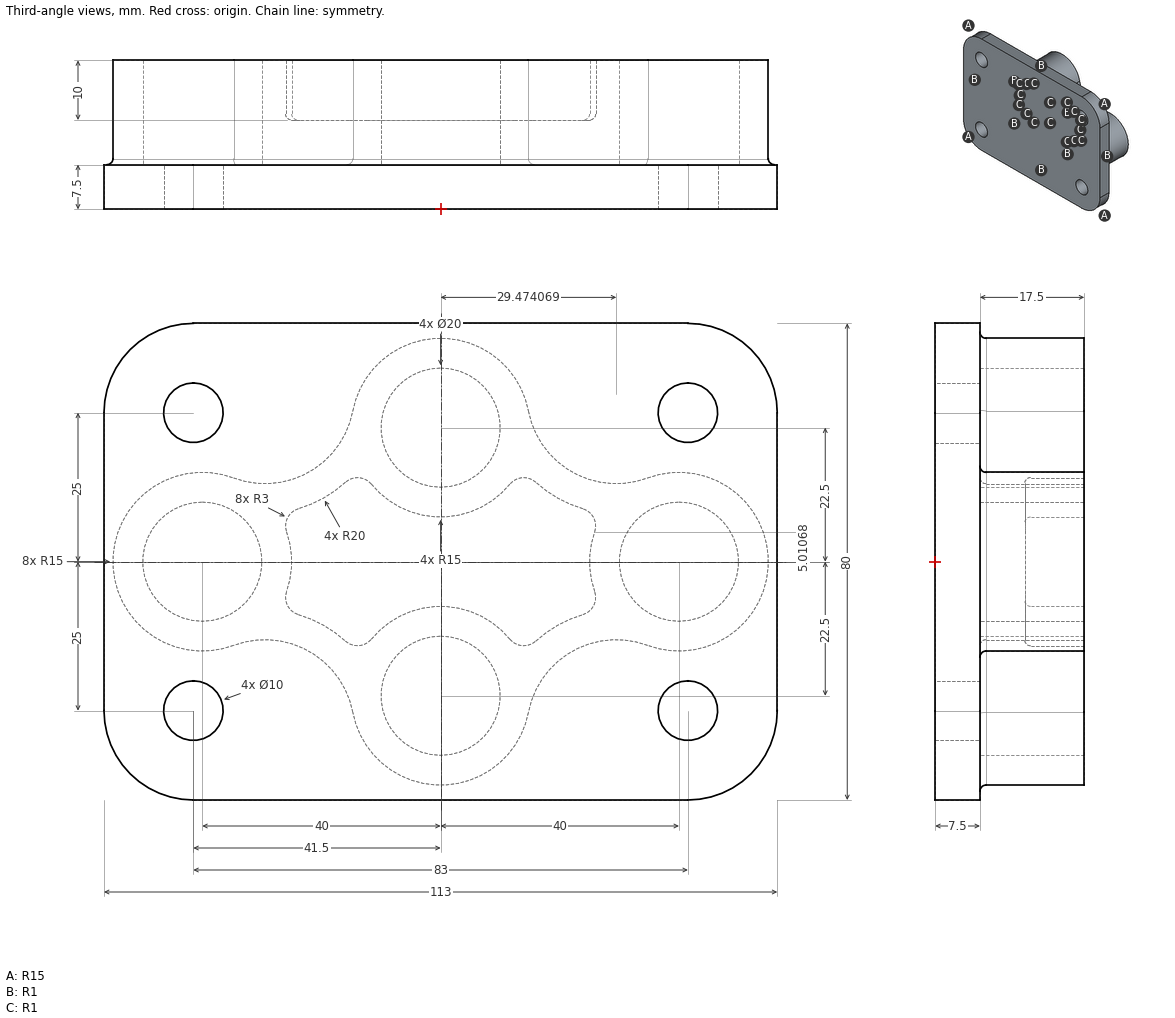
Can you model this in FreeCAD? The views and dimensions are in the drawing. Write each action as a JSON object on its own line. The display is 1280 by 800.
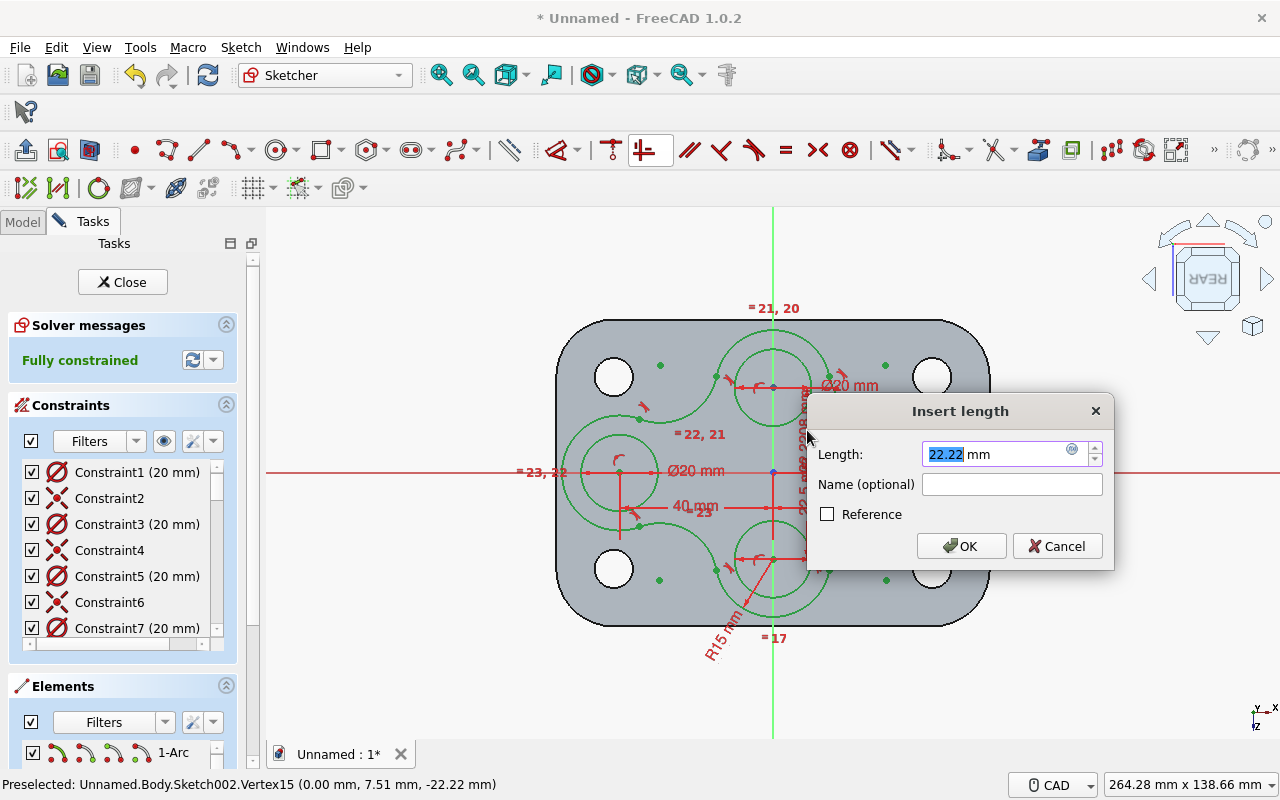
{"action": "type", "text": "22.5"}
{"action": "key", "text": "Return"}
{"action": "key", "text": "Escape"}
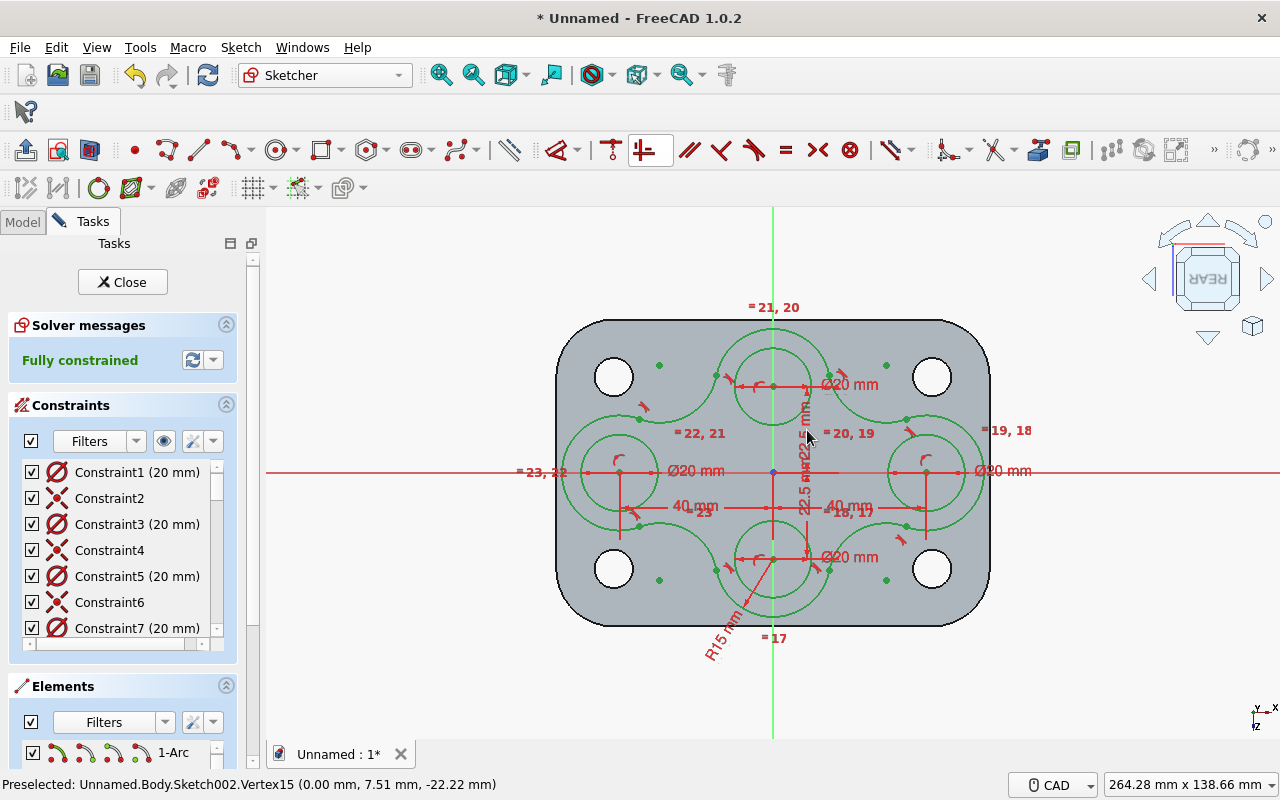
{"action": "left_click", "coordinate": [123, 282]}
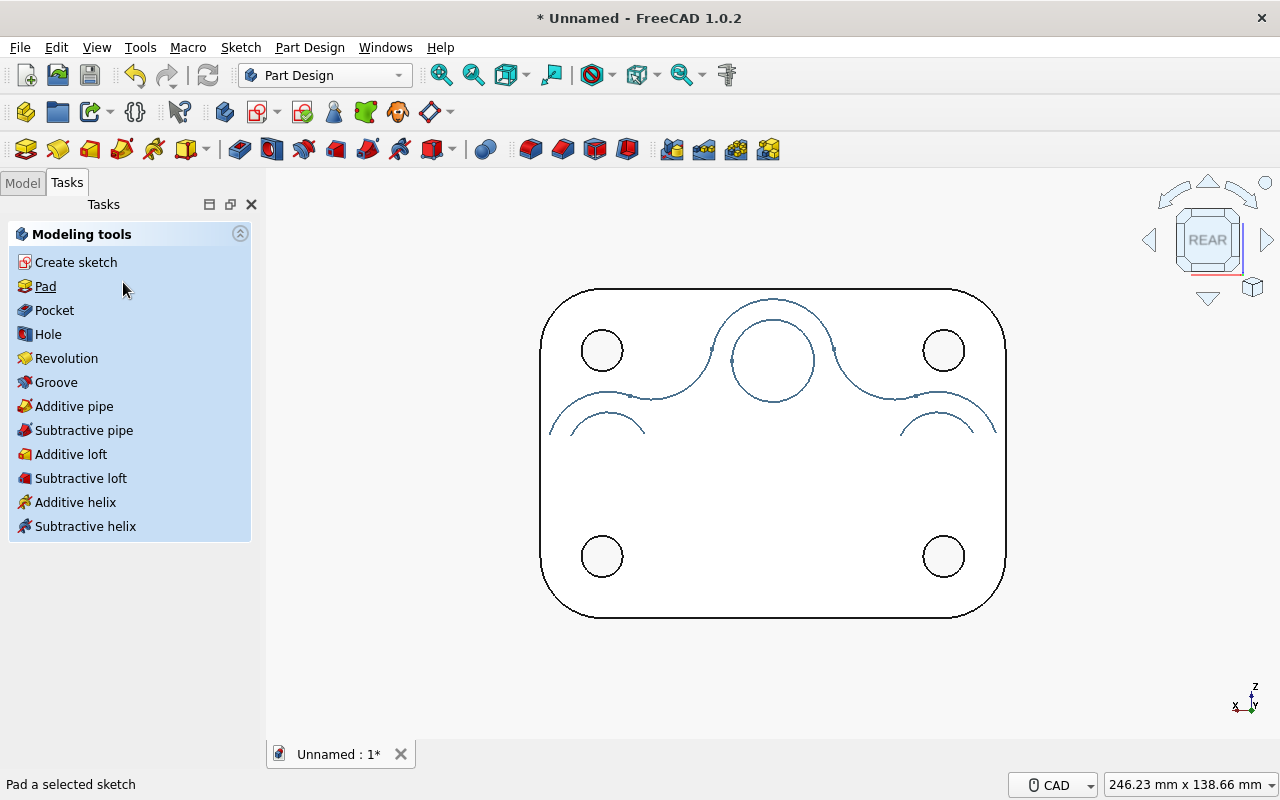
{"action": "left_click", "coordinate": [26, 150]}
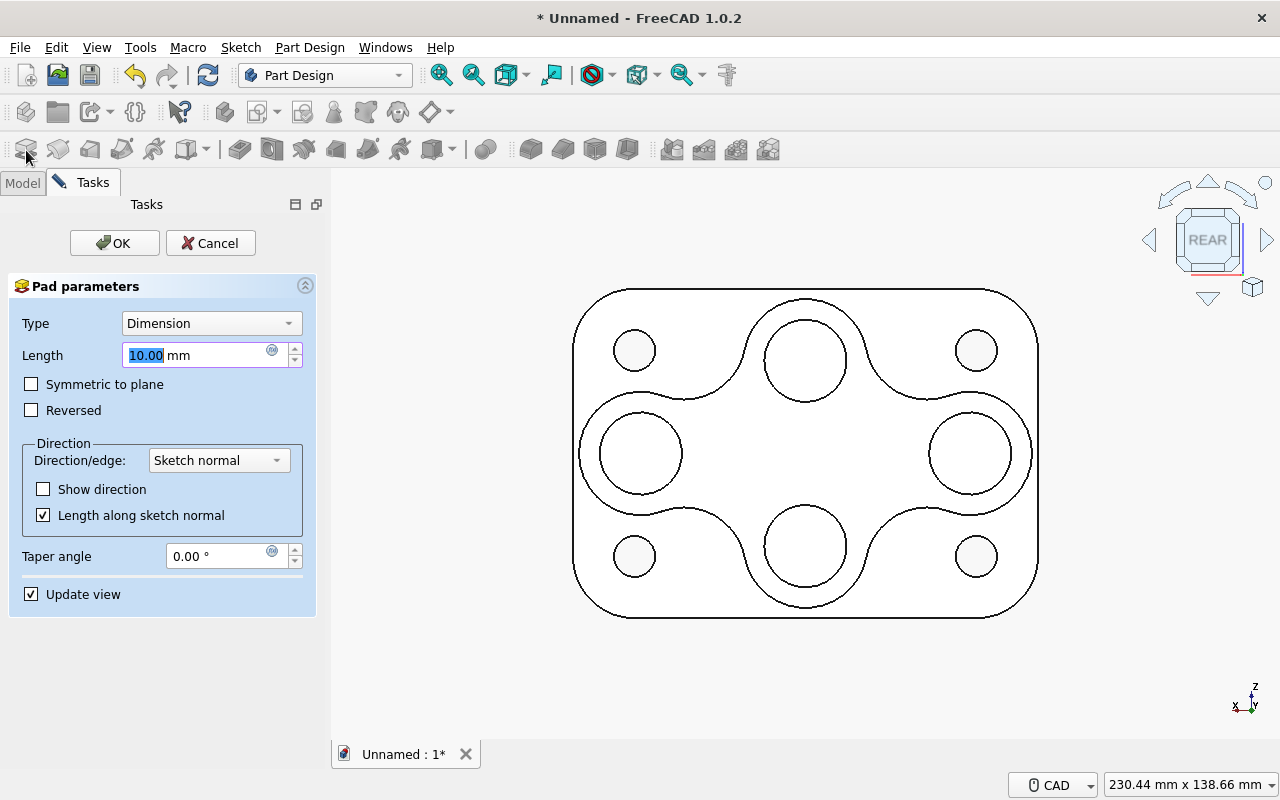
{"action": "type", "text": "17.5"}
{"action": "key", "text": "Tab"}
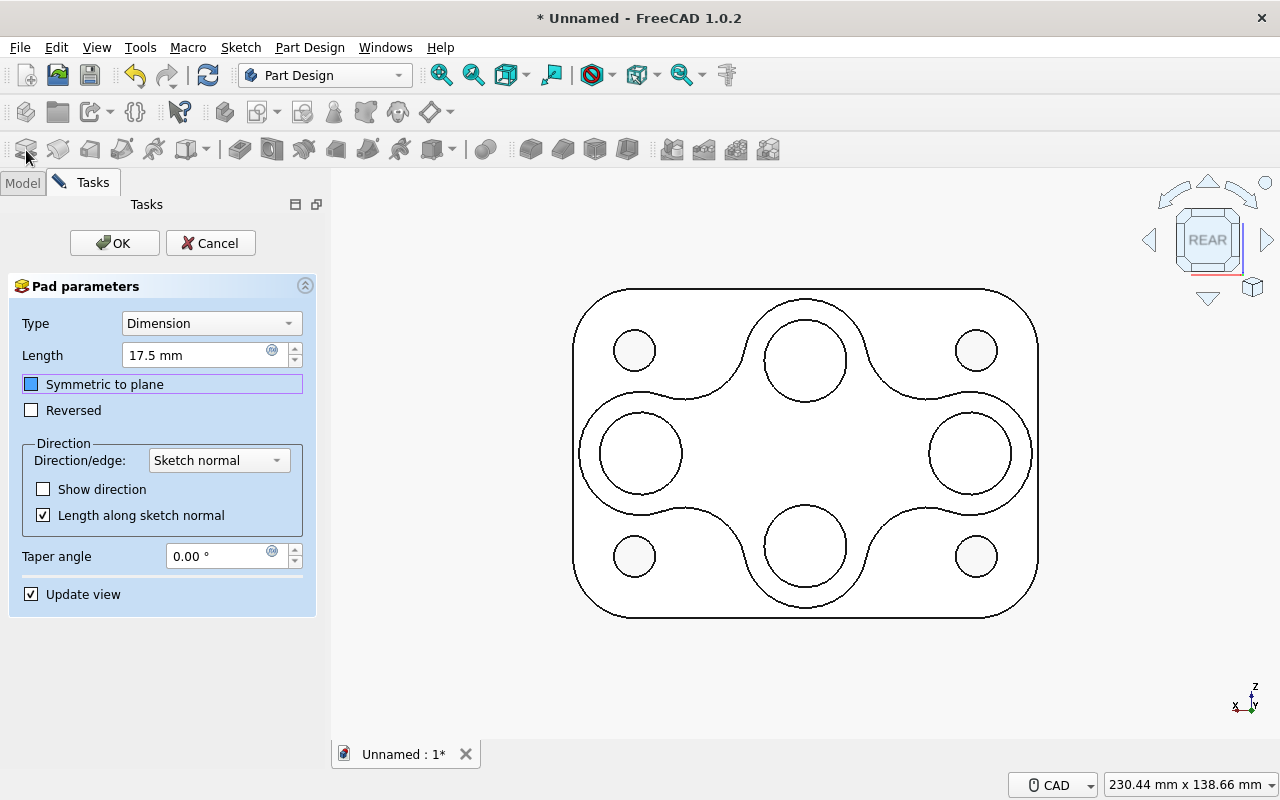
{"action": "left_click", "coordinate": [115, 243]}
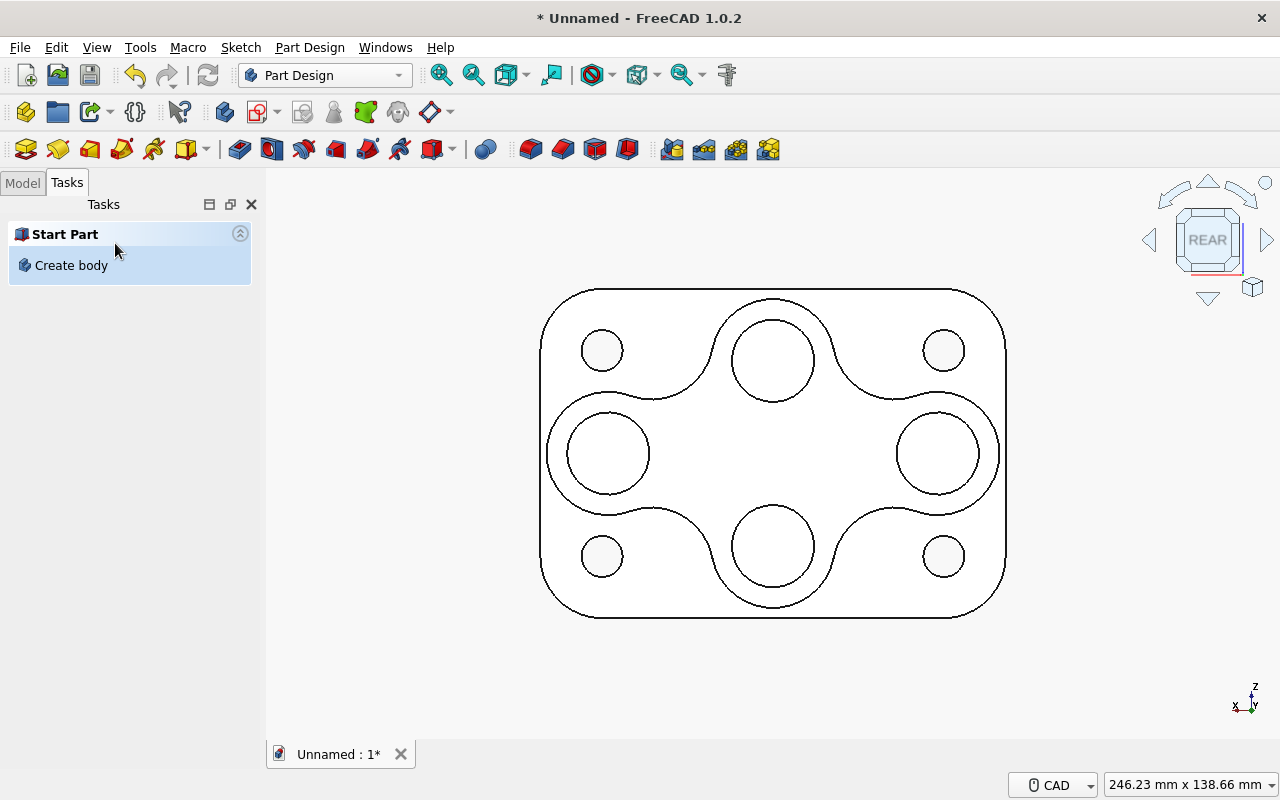
{"action": "left_click", "coordinate": [23, 182]}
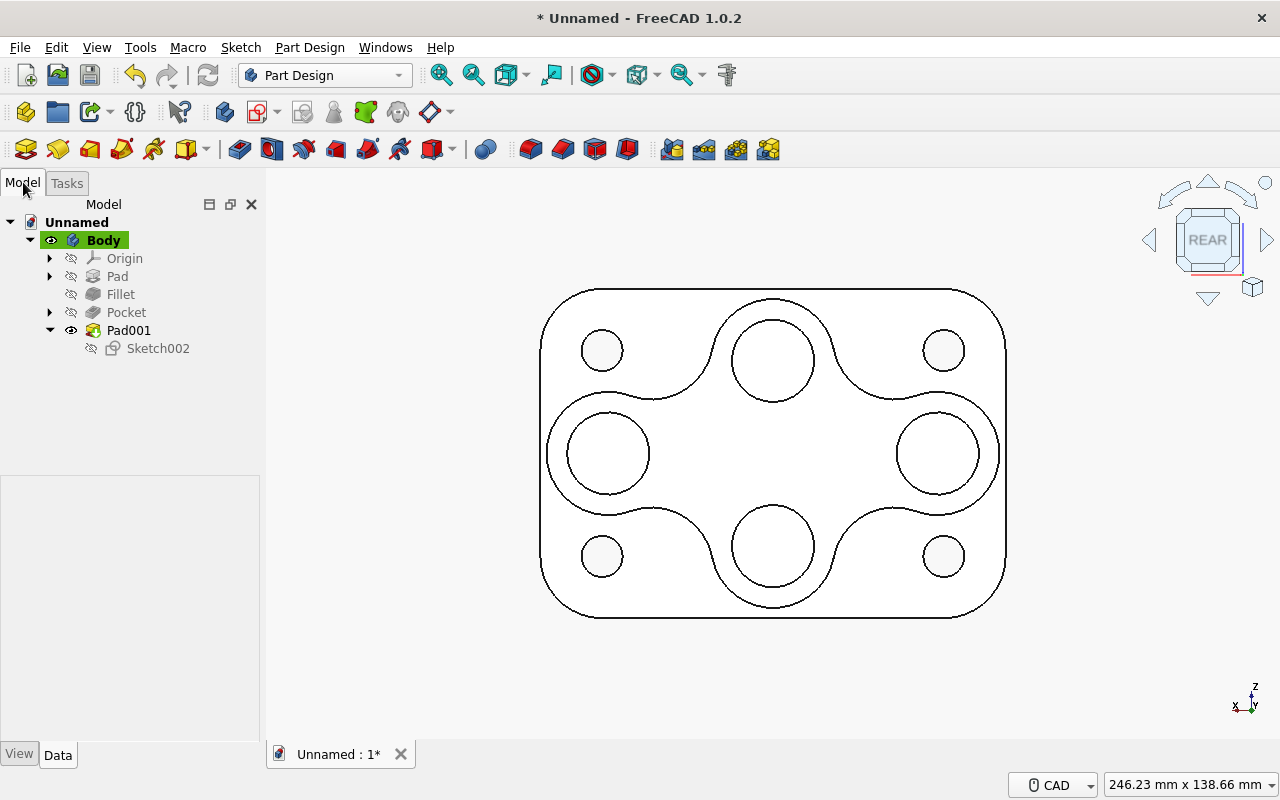
{"action": "left_click", "coordinate": [50, 258]}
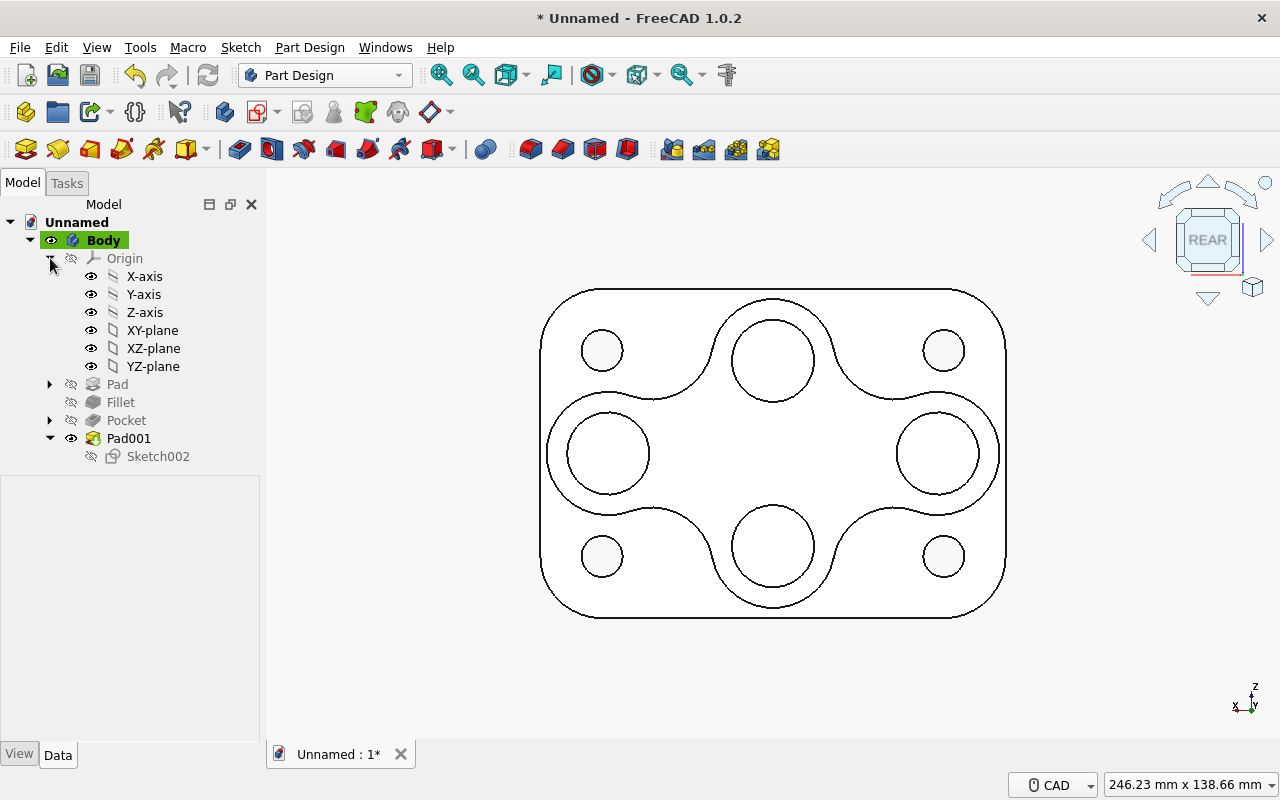
{"action": "left_click", "coordinate": [136, 348]}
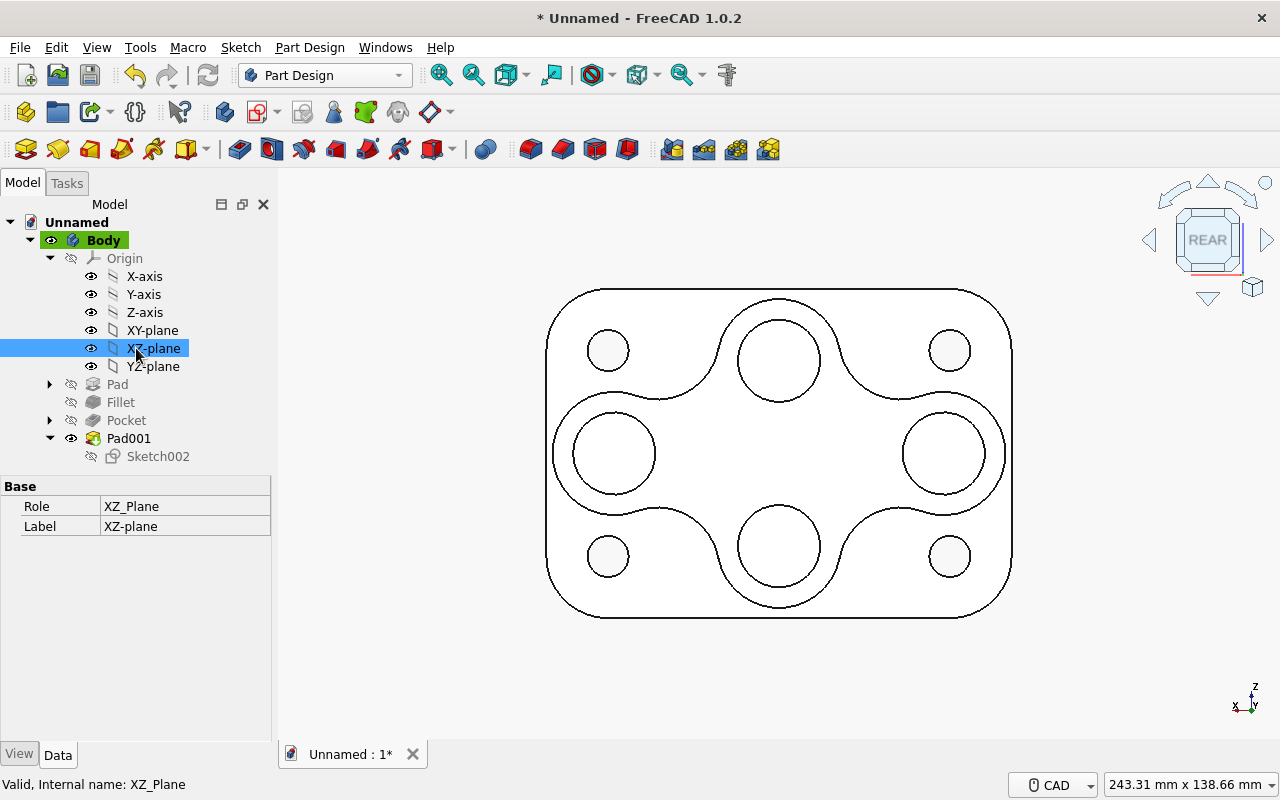
{"action": "left_click", "coordinate": [430, 112]}